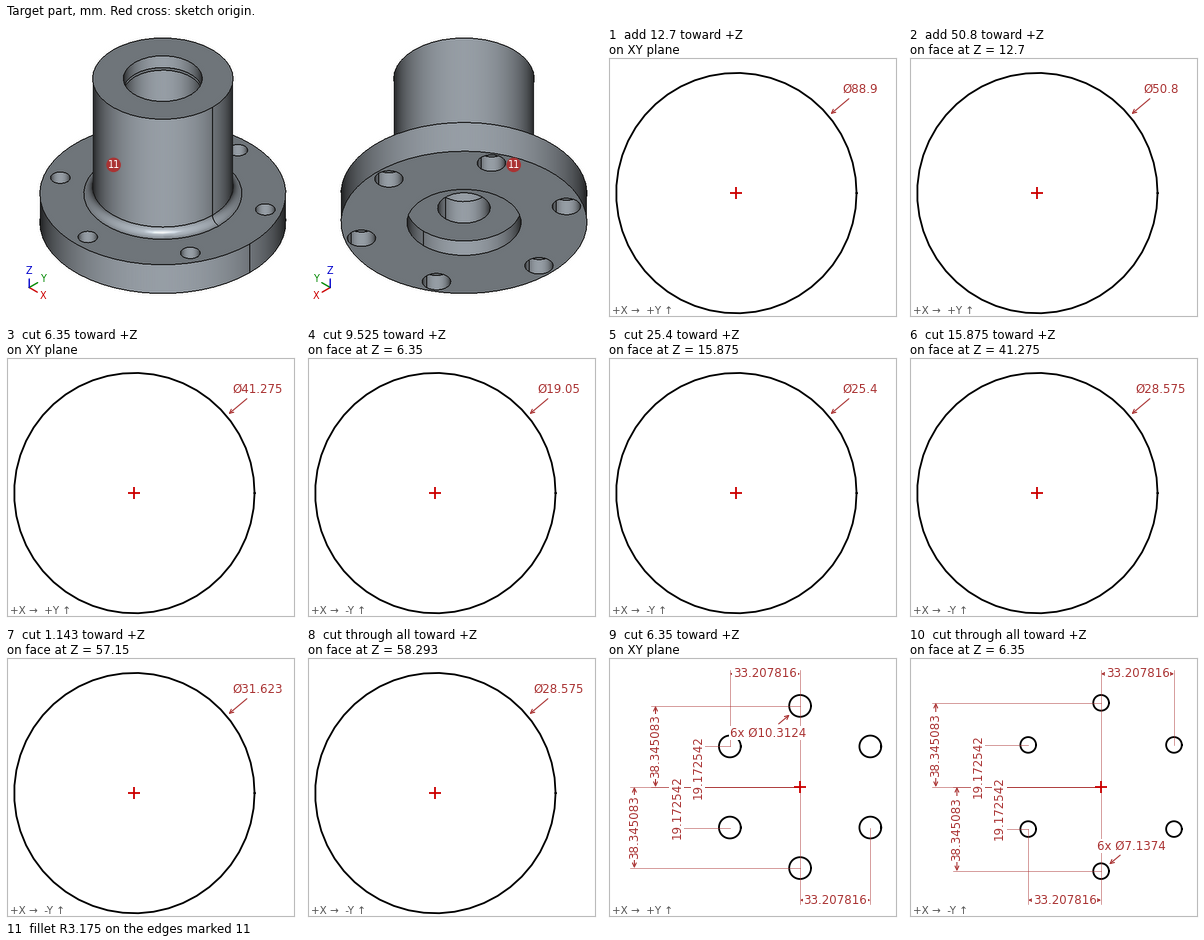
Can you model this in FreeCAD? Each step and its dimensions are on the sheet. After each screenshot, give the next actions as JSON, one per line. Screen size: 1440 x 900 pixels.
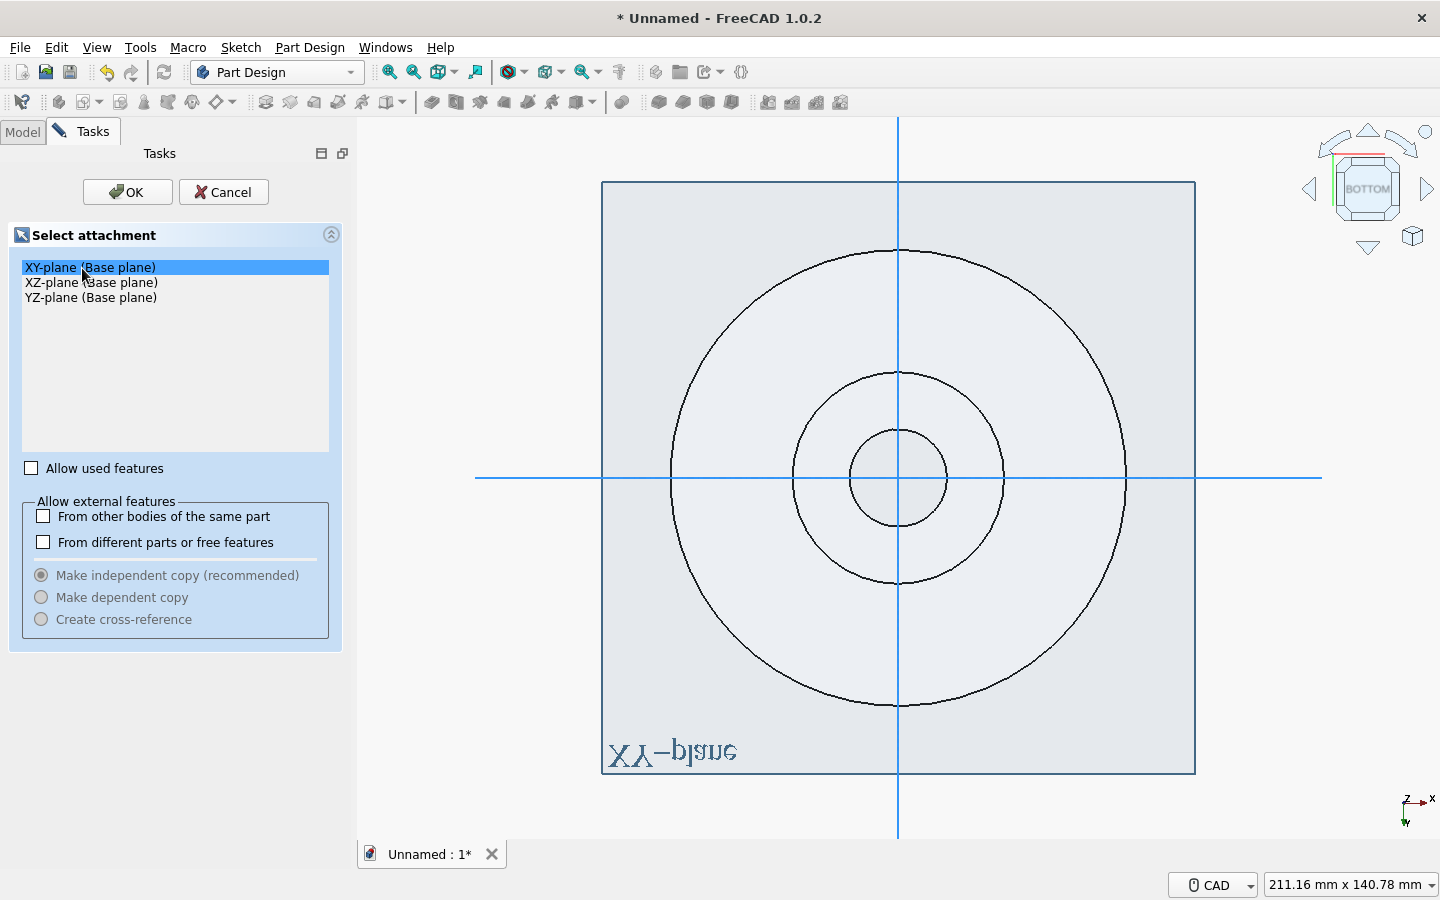
{"action": "left_click", "coordinate": [128, 192]}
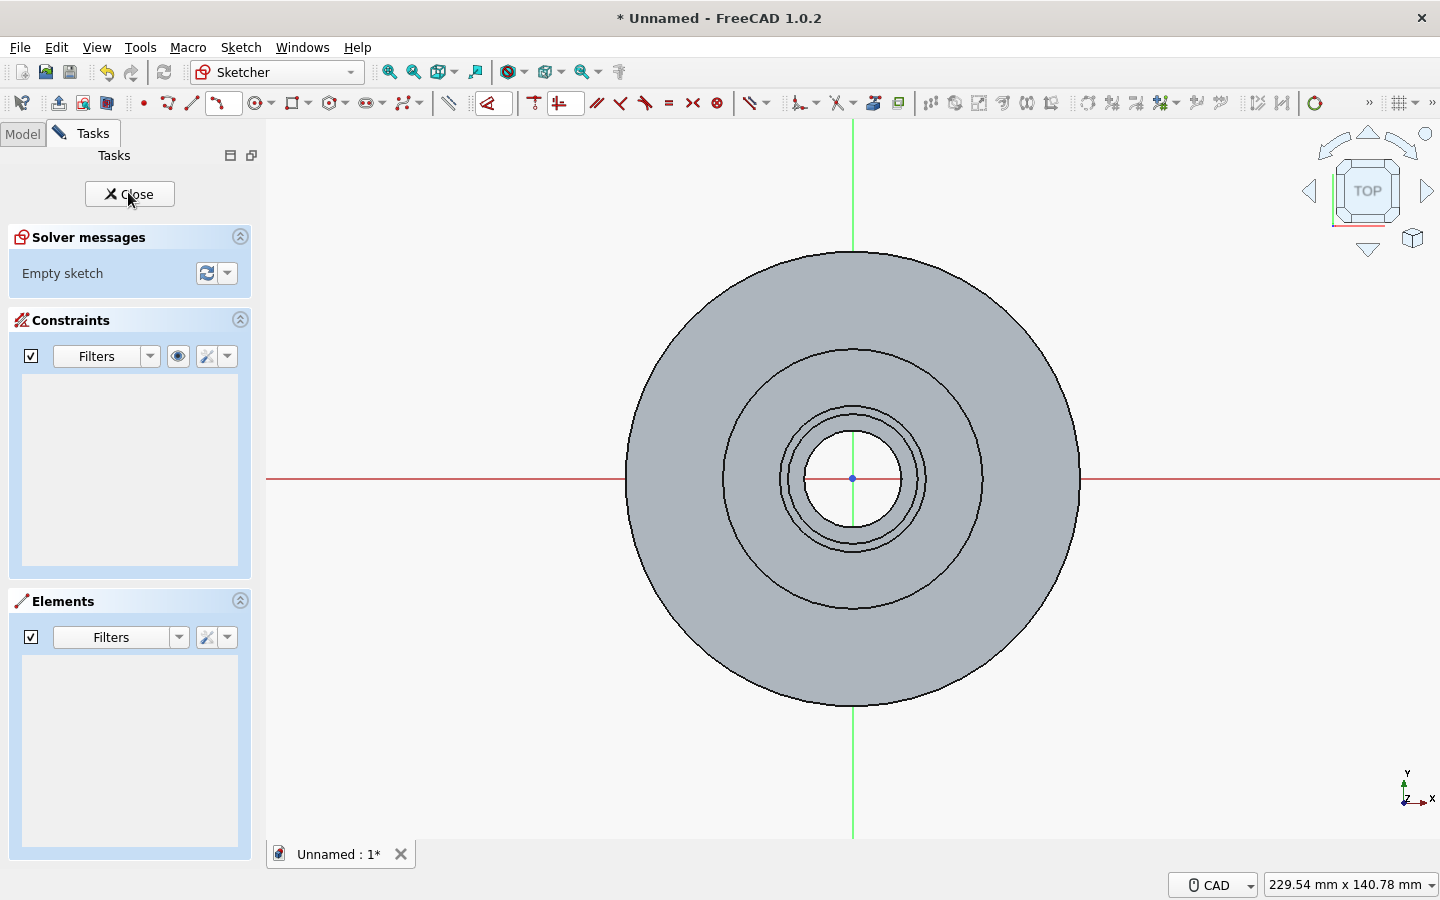
{"action": "left_click", "coordinate": [108, 104]}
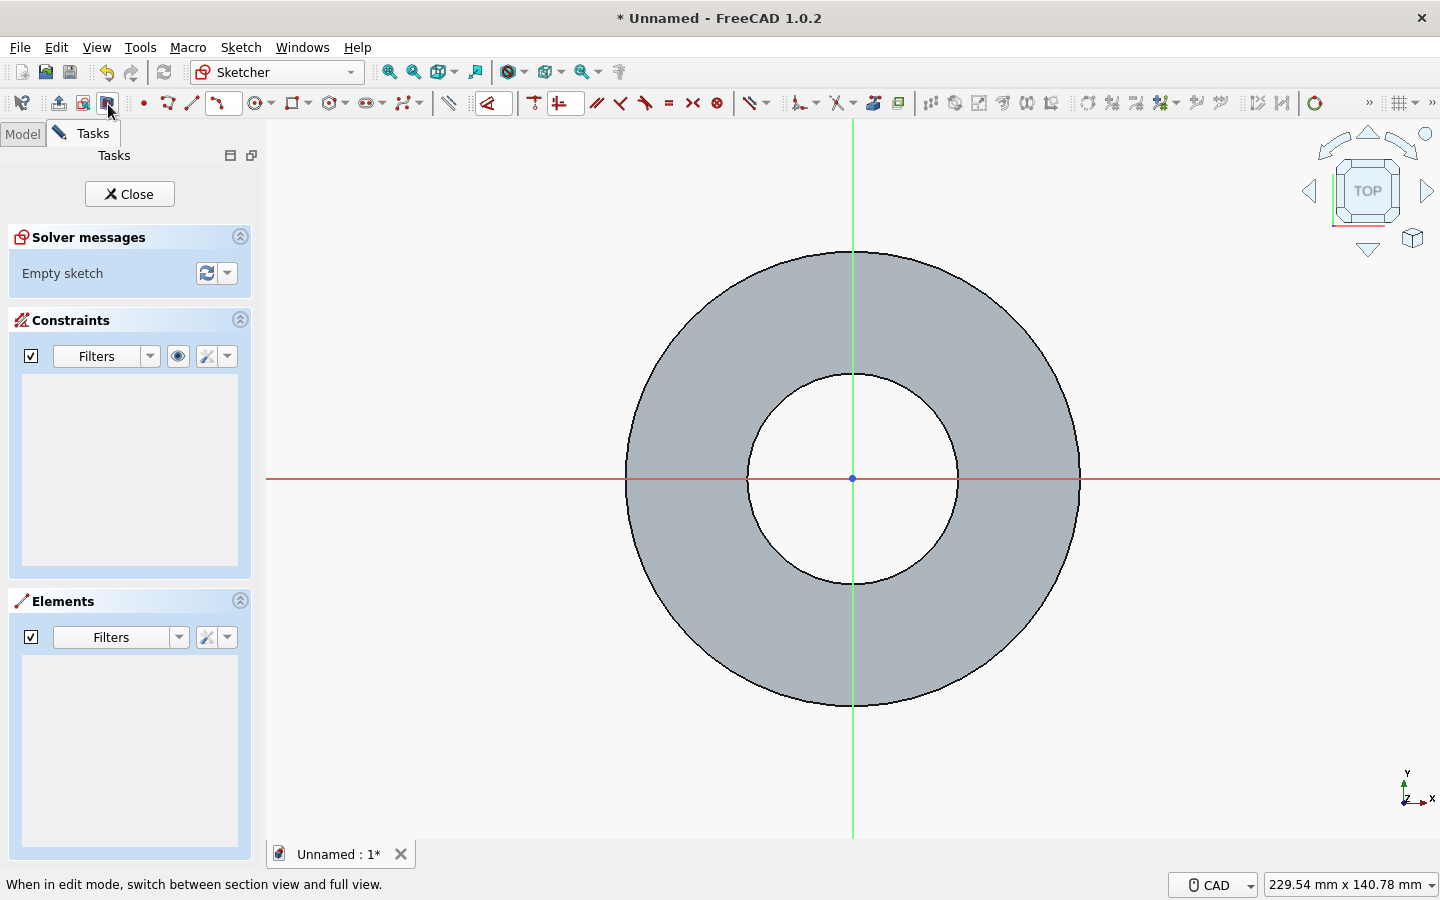
{"action": "left_click", "coordinate": [256, 104]}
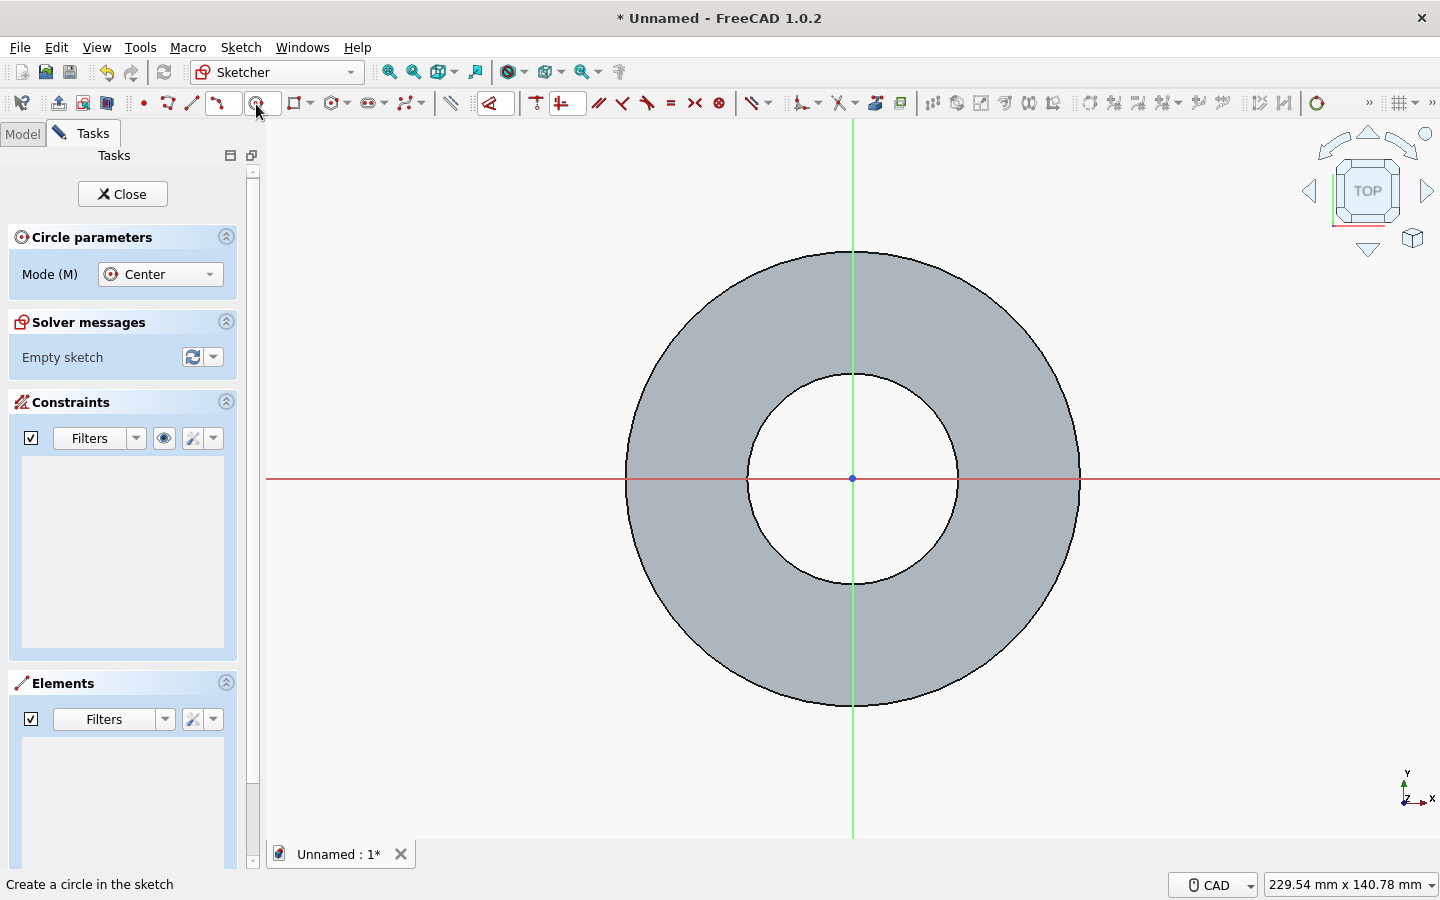
{"action": "left_click", "coordinate": [853, 283]}
{"action": "mouse_move", "coordinate": [871, 264]}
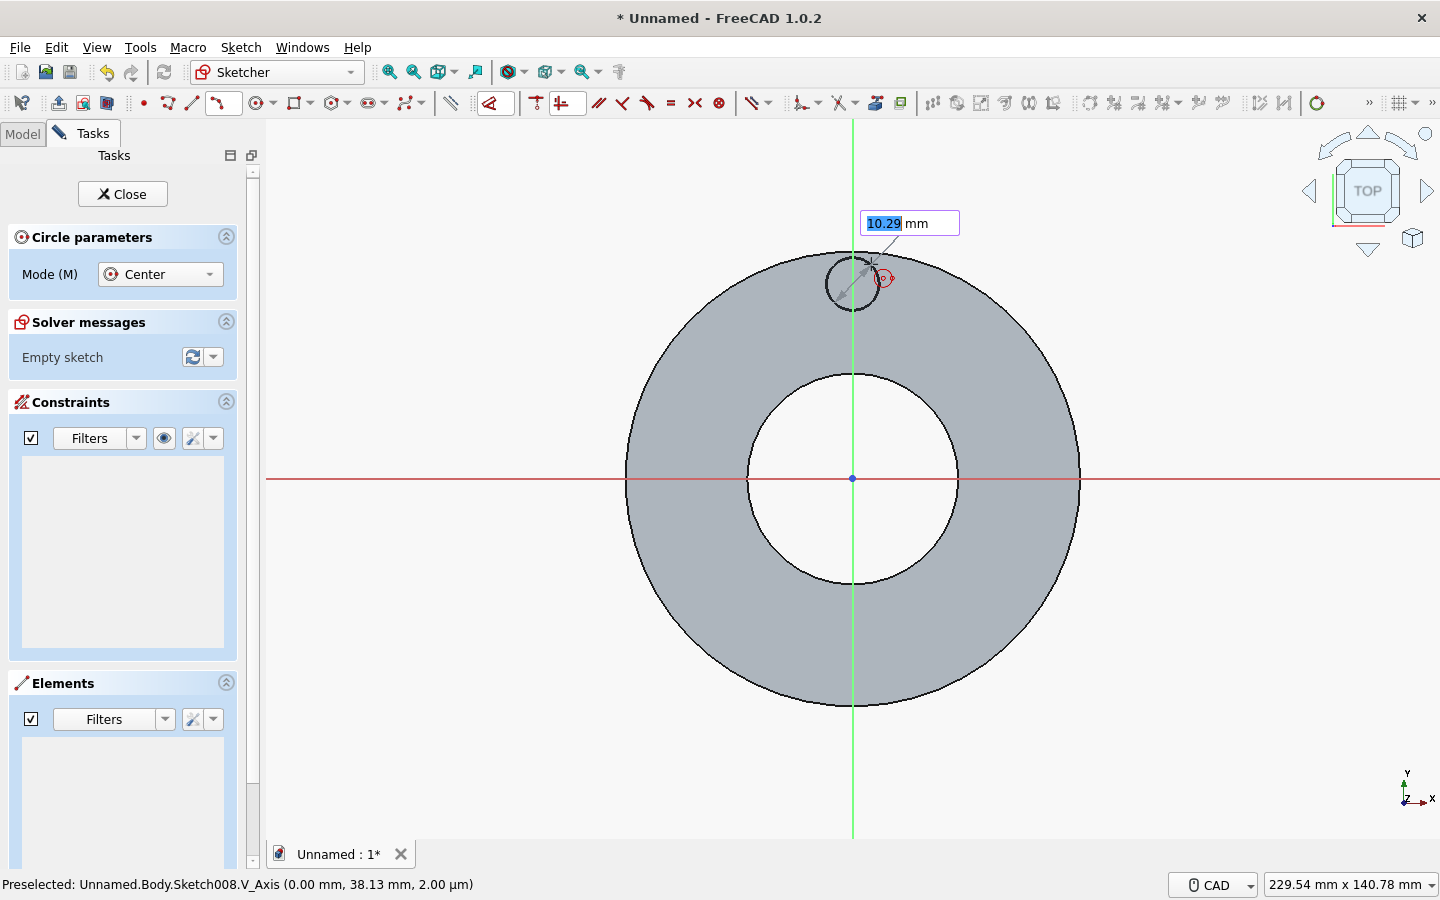
{"action": "type", "text": "10.3124"}
{"action": "key", "text": "Return"}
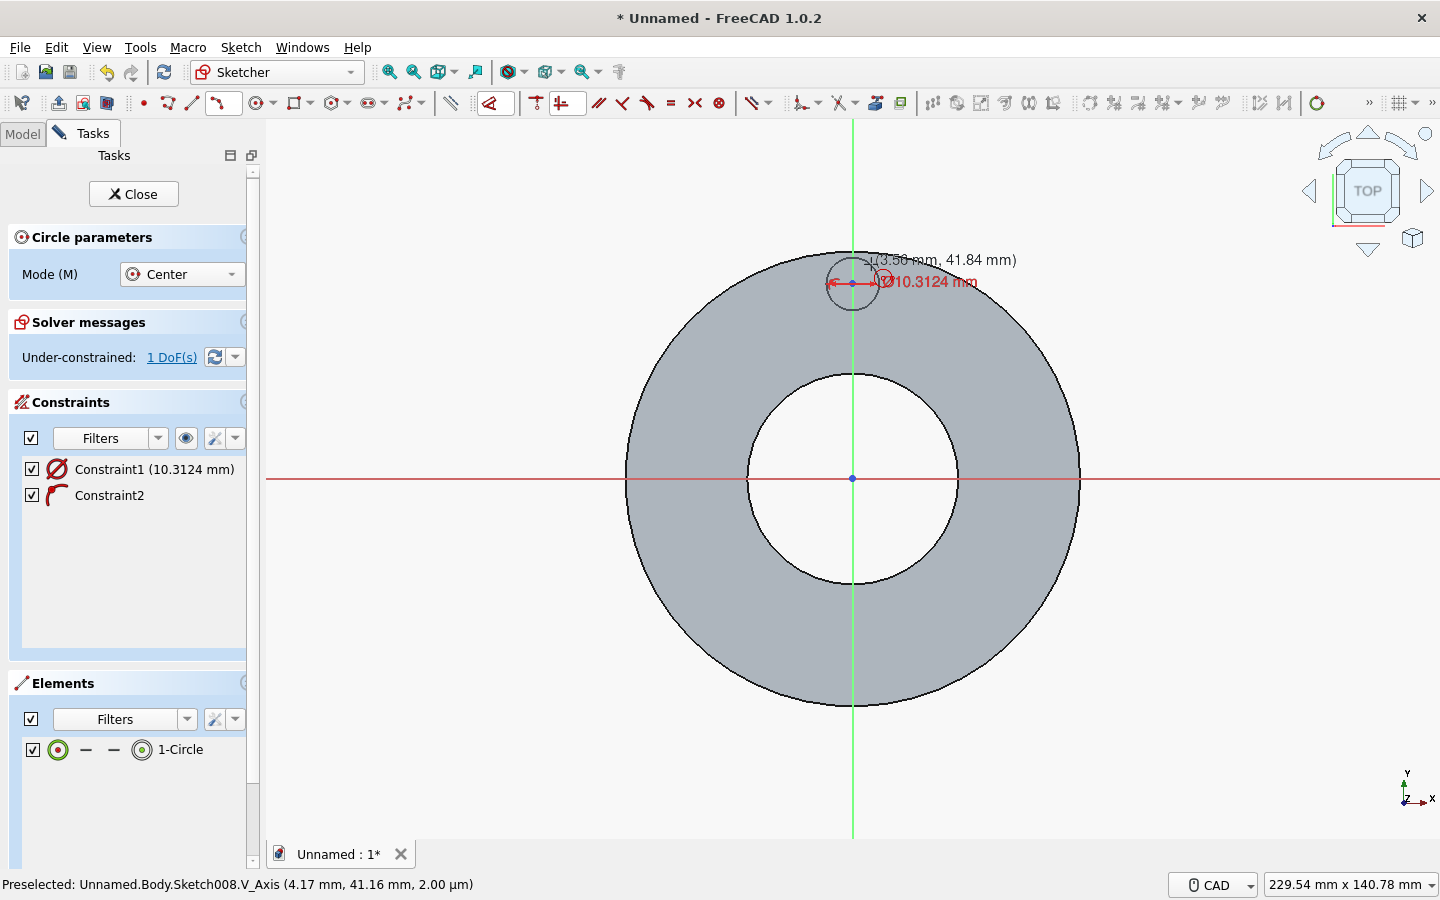
{"action": "left_click", "coordinate": [683, 381]}
{"action": "mouse_move", "coordinate": [702, 362]}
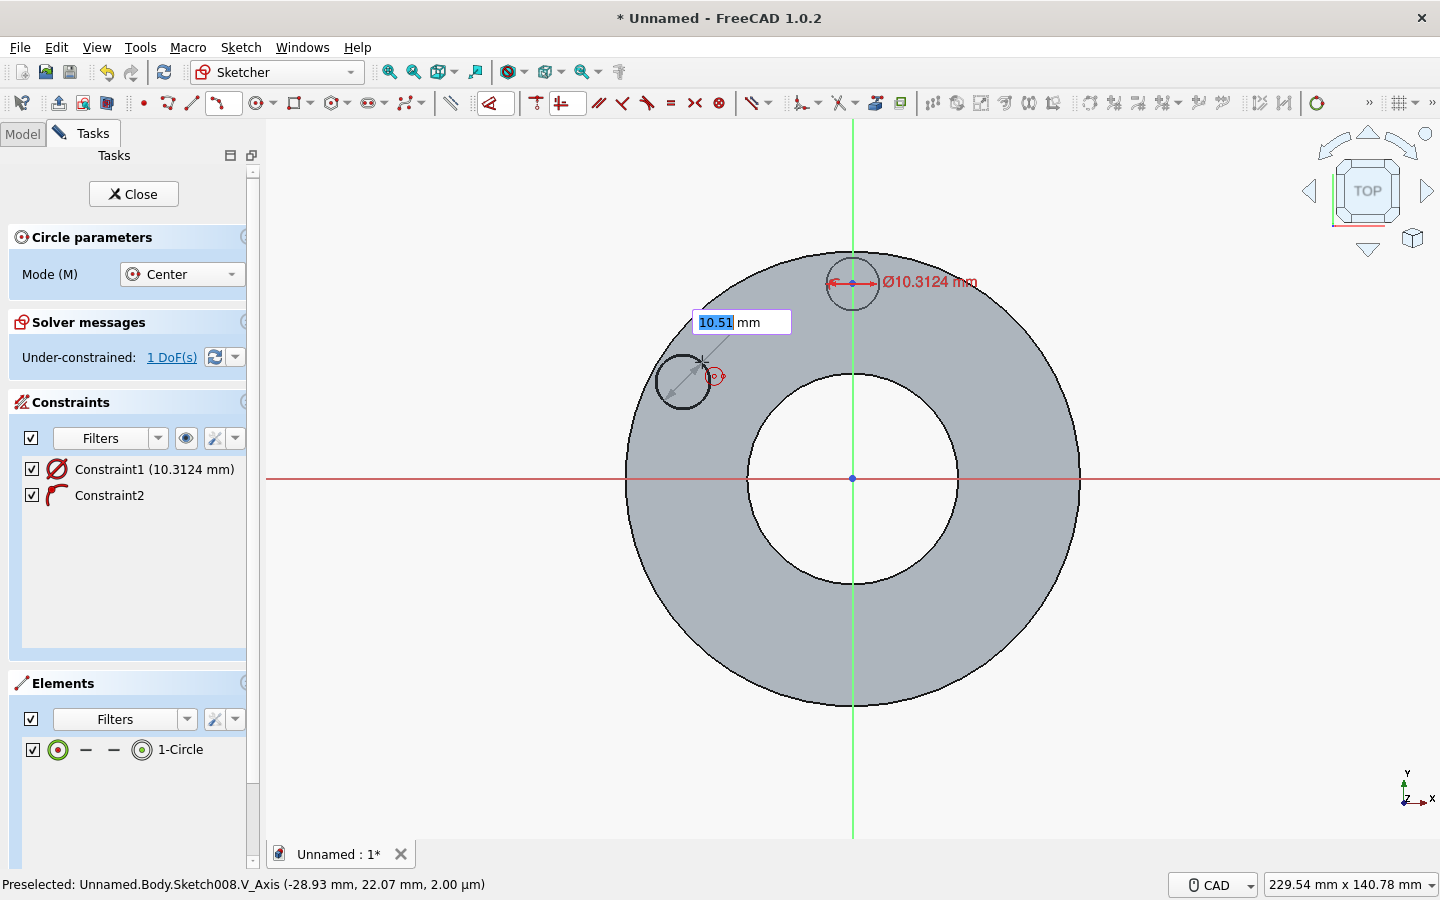
{"action": "type", "text": "10.3124"}
{"action": "key", "text": "Return"}